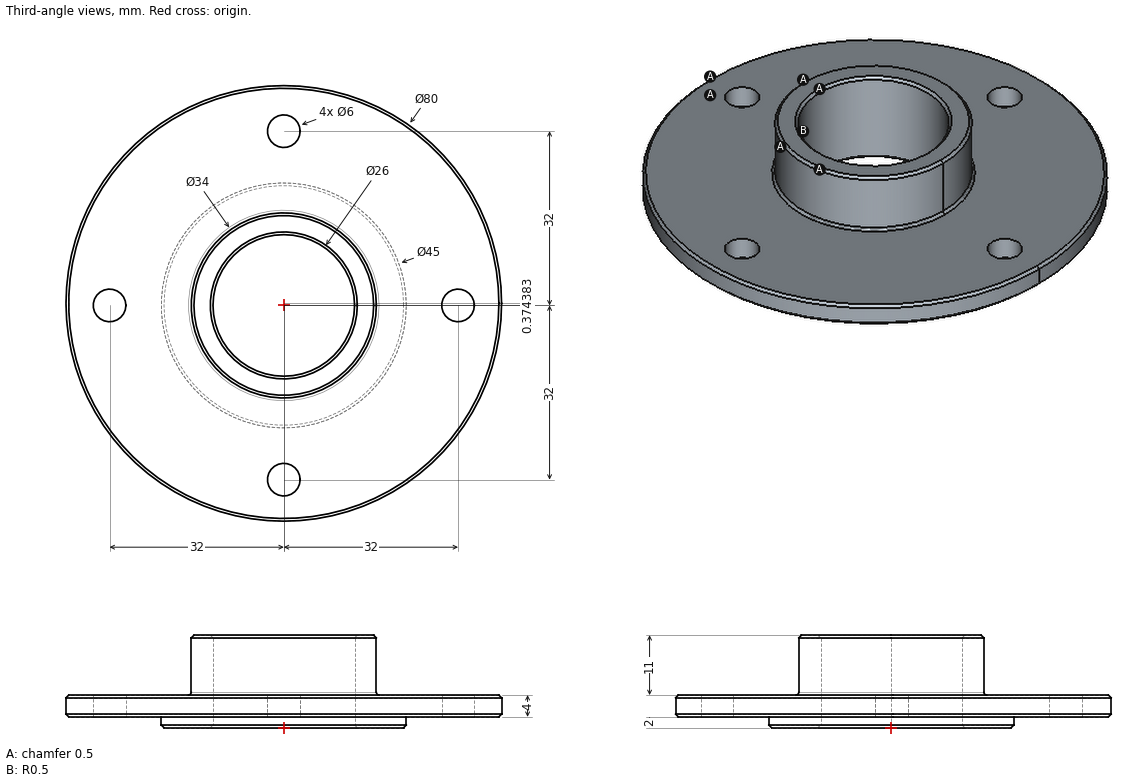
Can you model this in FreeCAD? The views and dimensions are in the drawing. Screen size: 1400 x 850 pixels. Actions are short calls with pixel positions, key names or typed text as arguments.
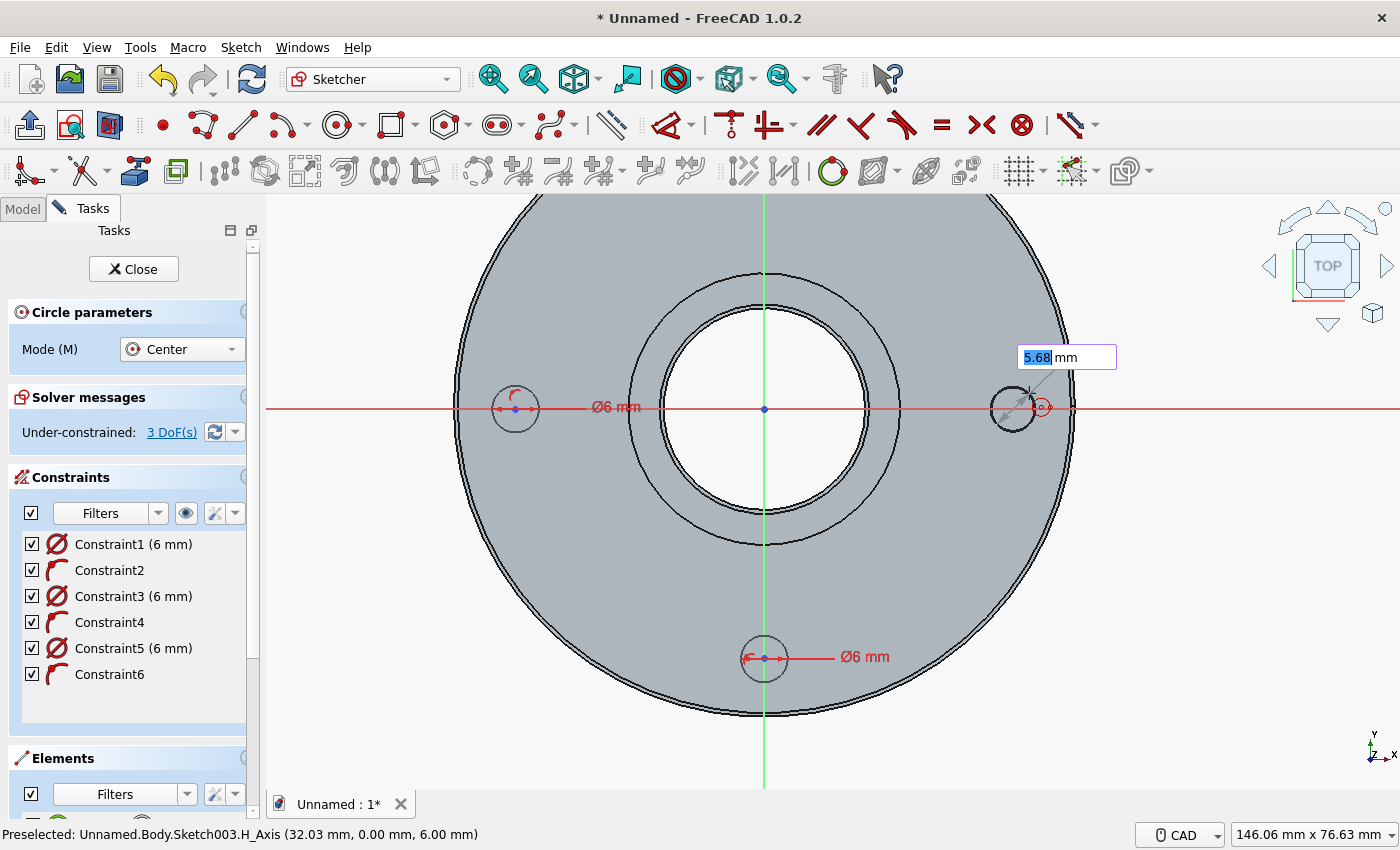
text(6)
key(Return)
key(Escape)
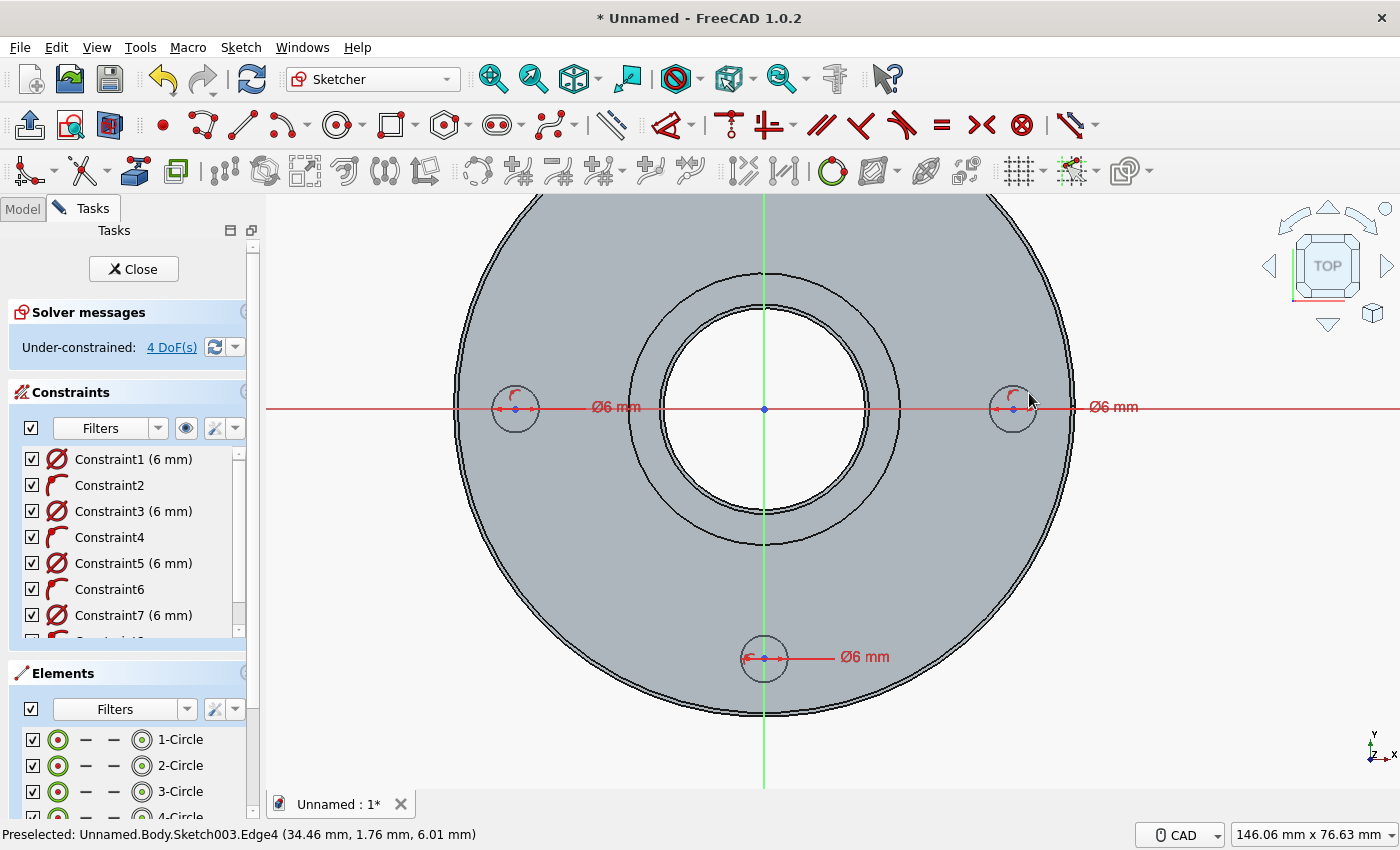
click(666, 126)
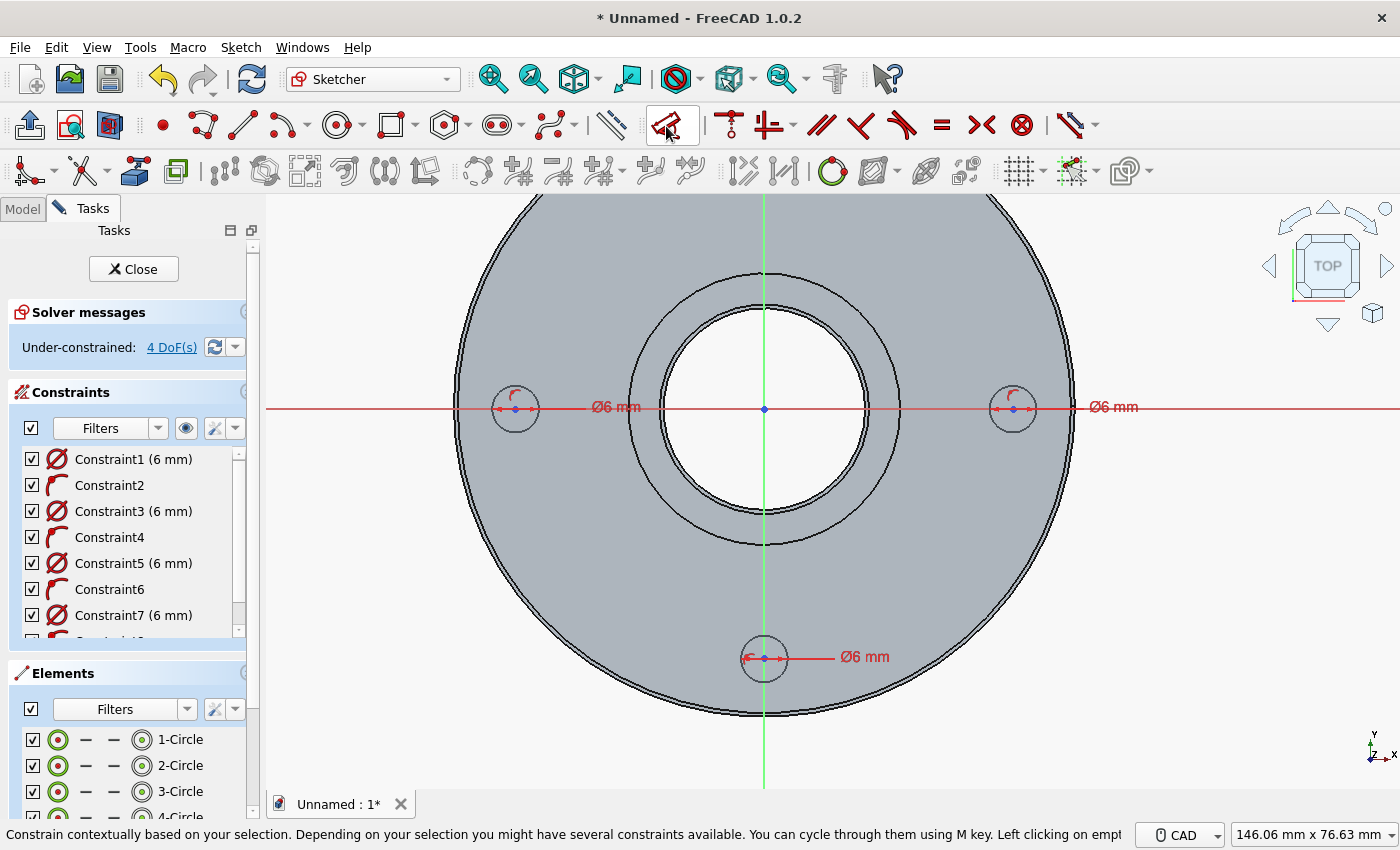
scroll(765, 659, down, 2)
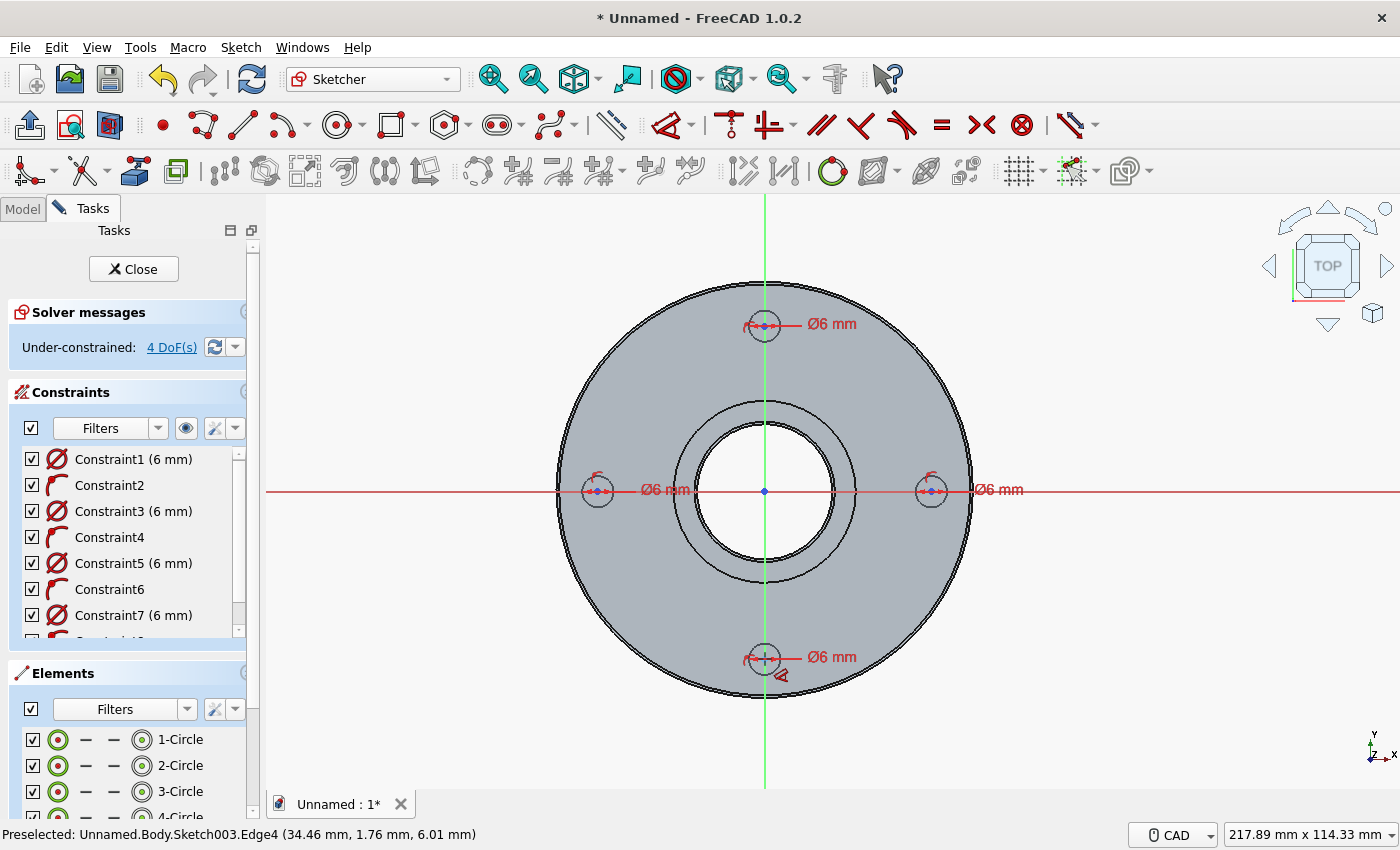
click(765, 326)
click(799, 409)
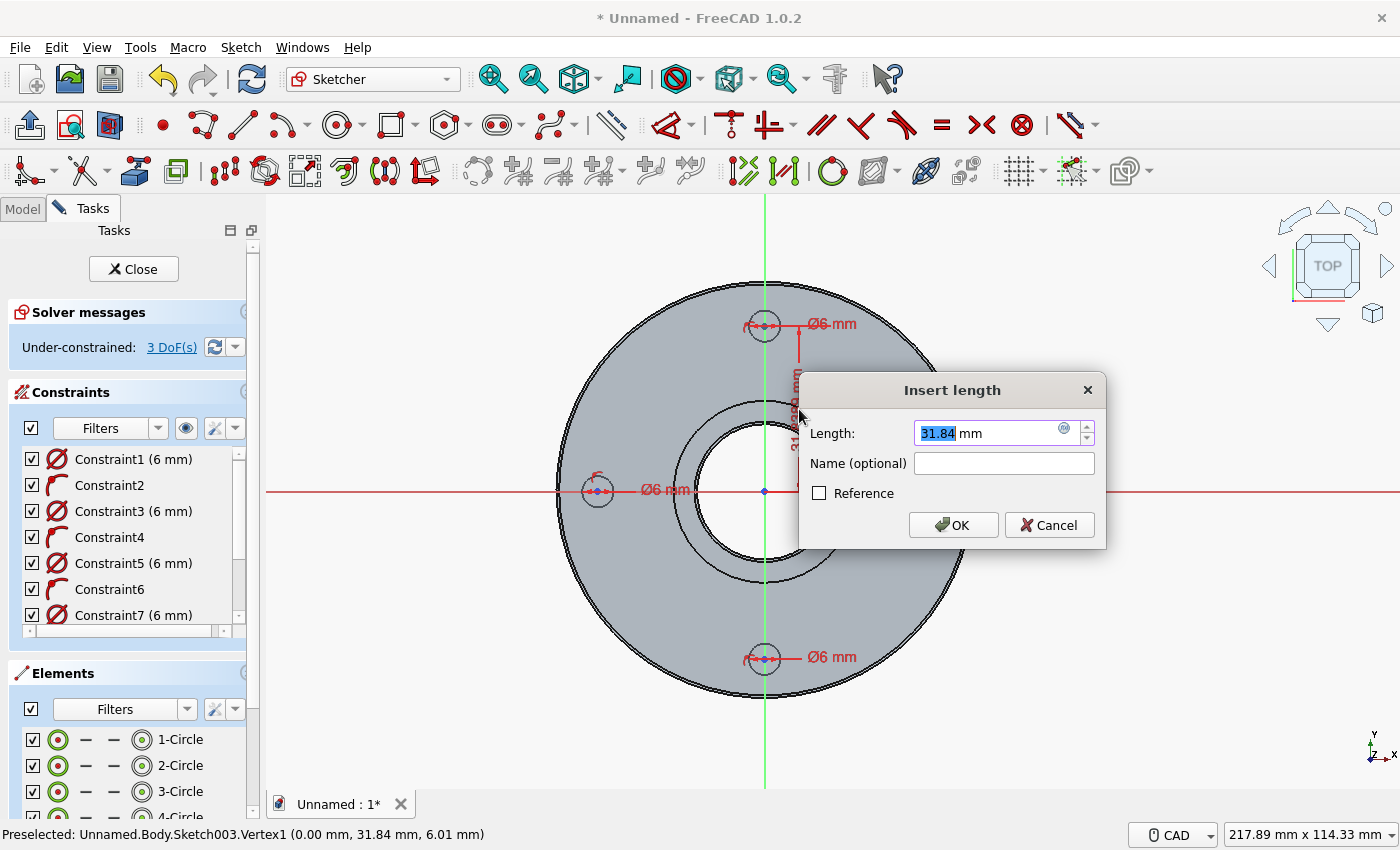
text(32)
key(Return)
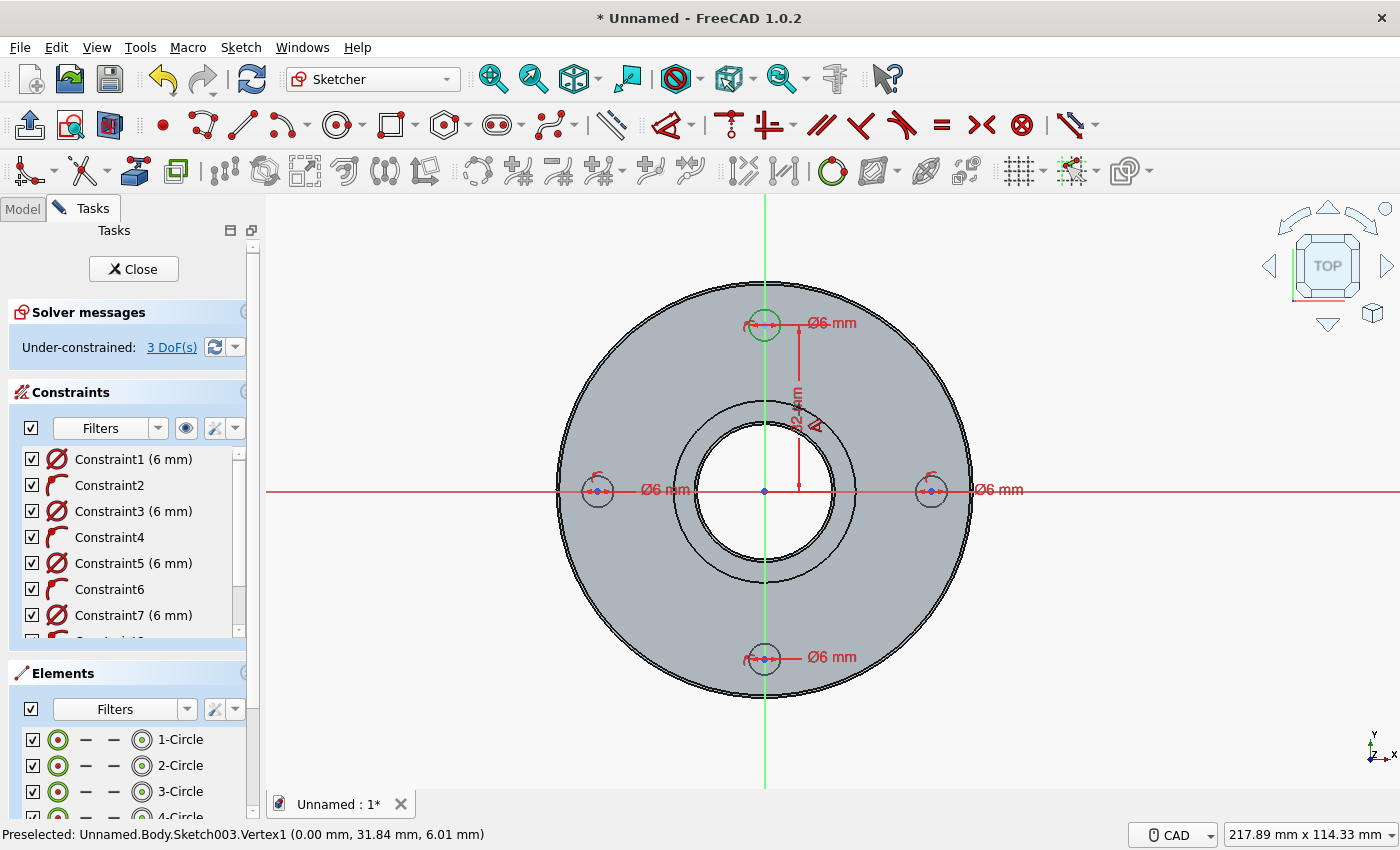
click(598, 492)
click(681, 526)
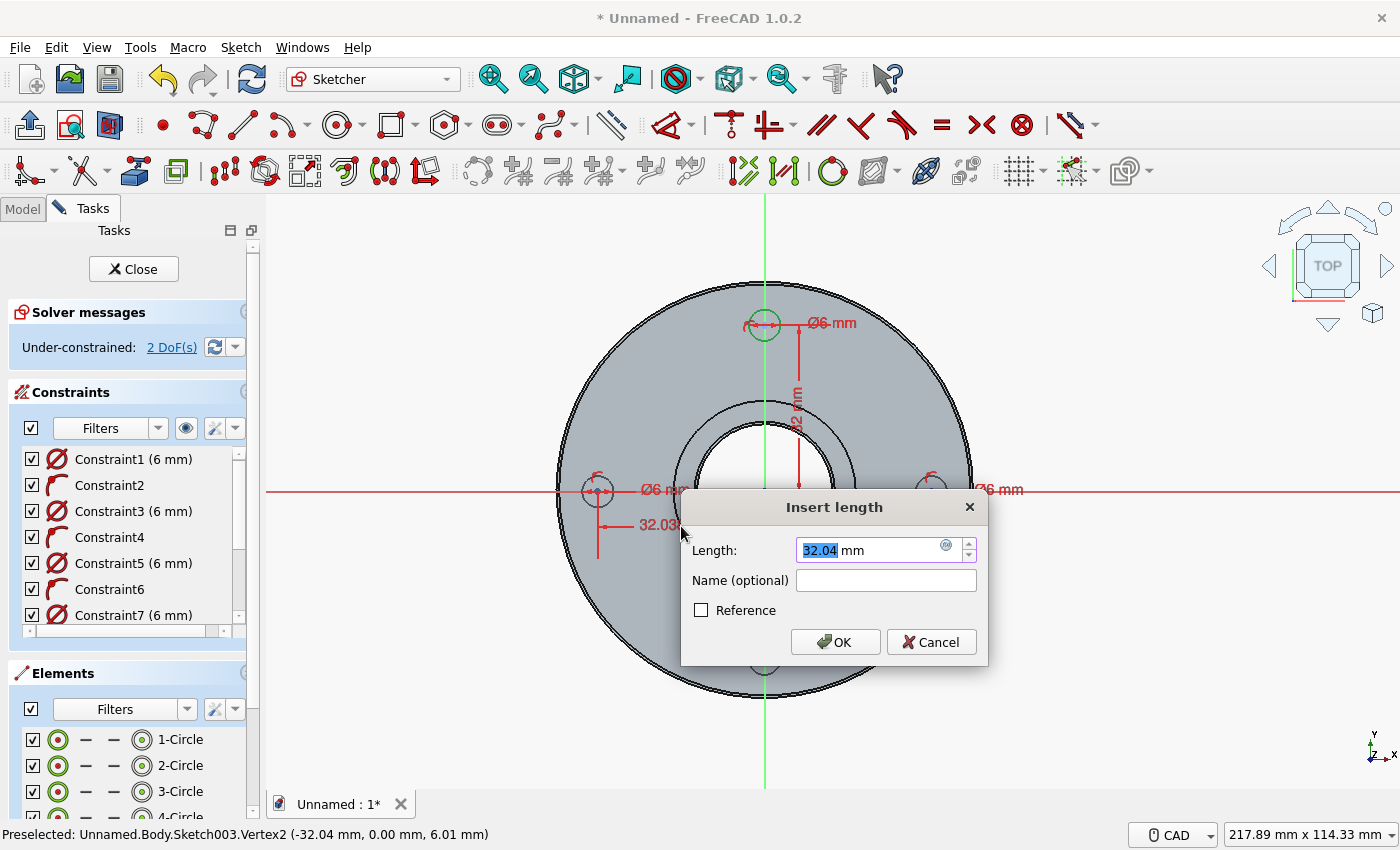
text(32)
key(Return)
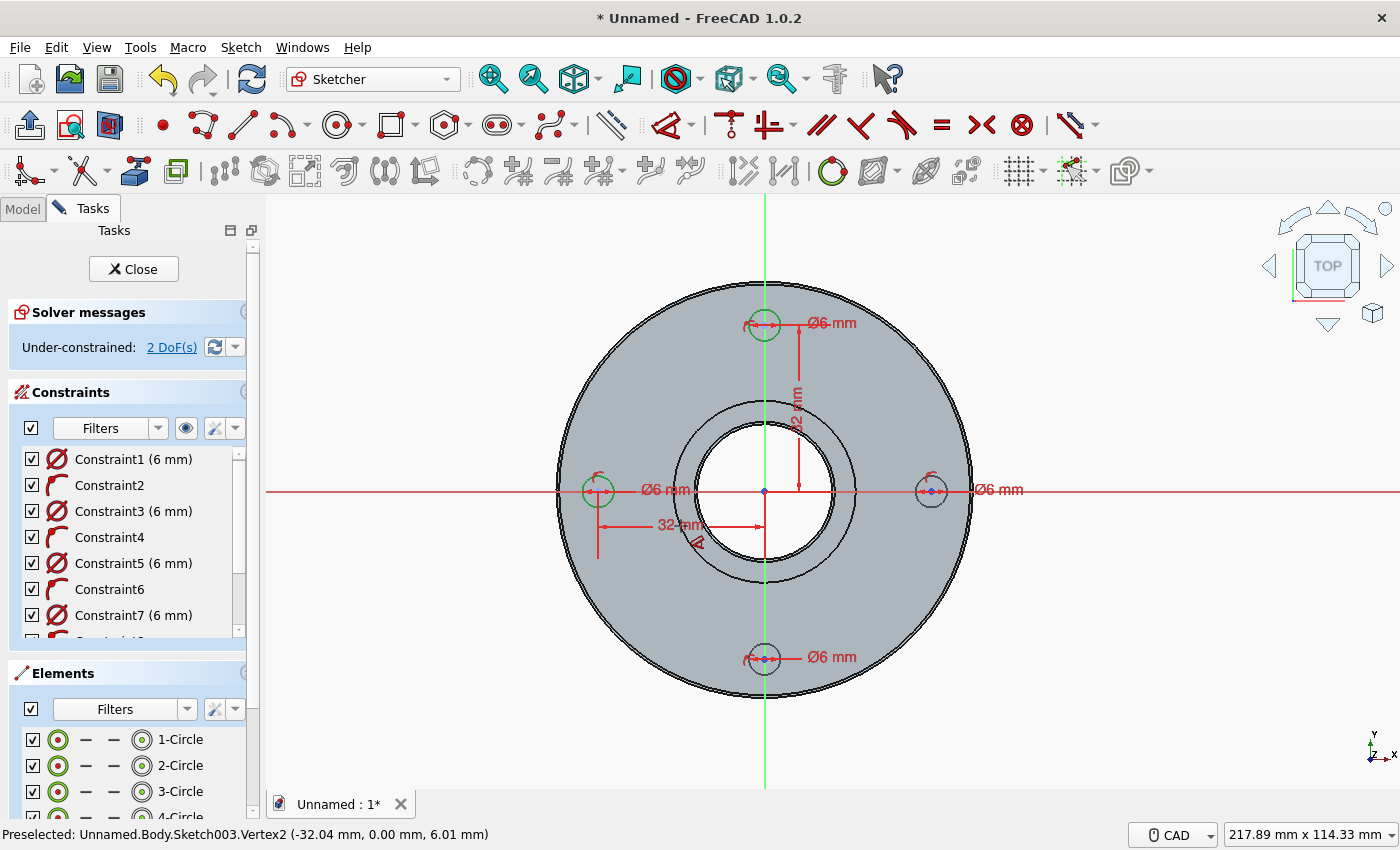
click(765, 659)
click(799, 576)